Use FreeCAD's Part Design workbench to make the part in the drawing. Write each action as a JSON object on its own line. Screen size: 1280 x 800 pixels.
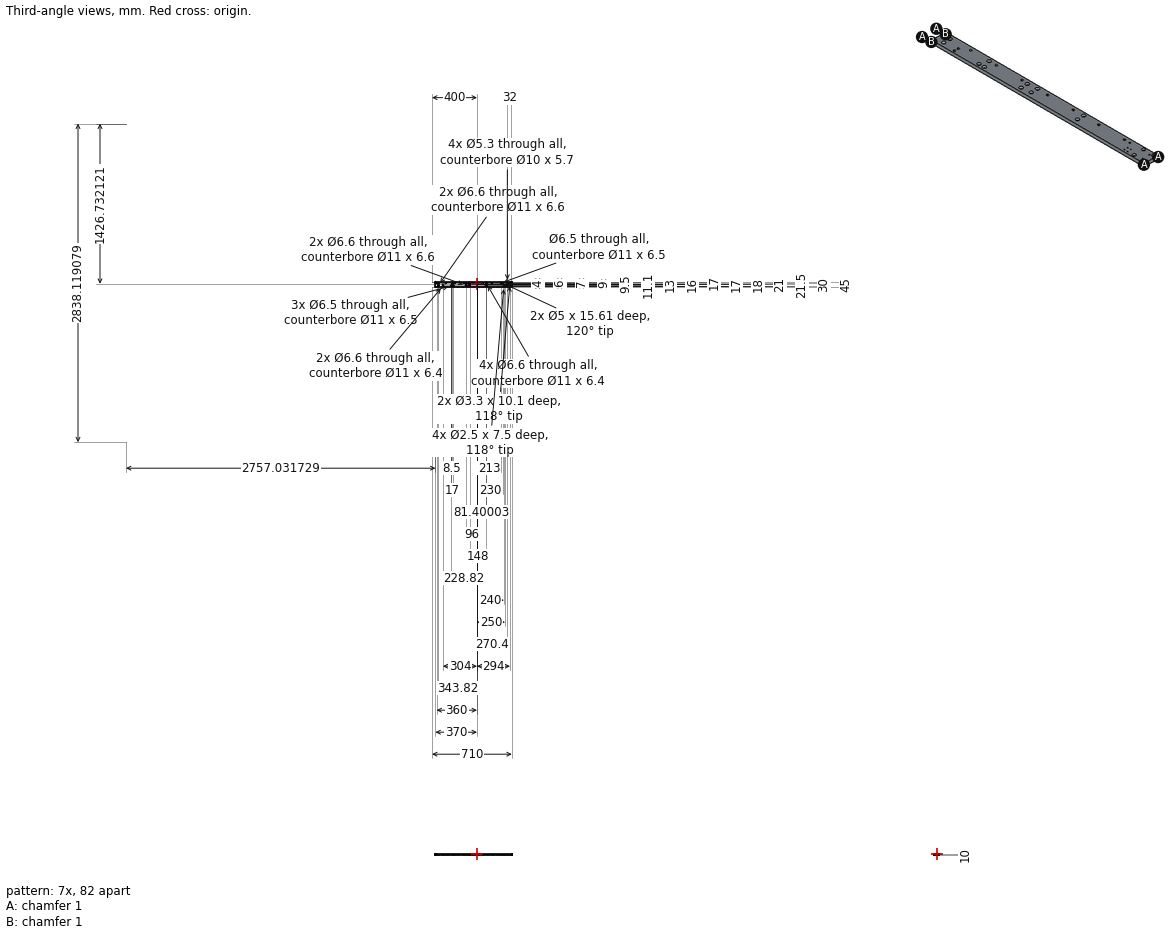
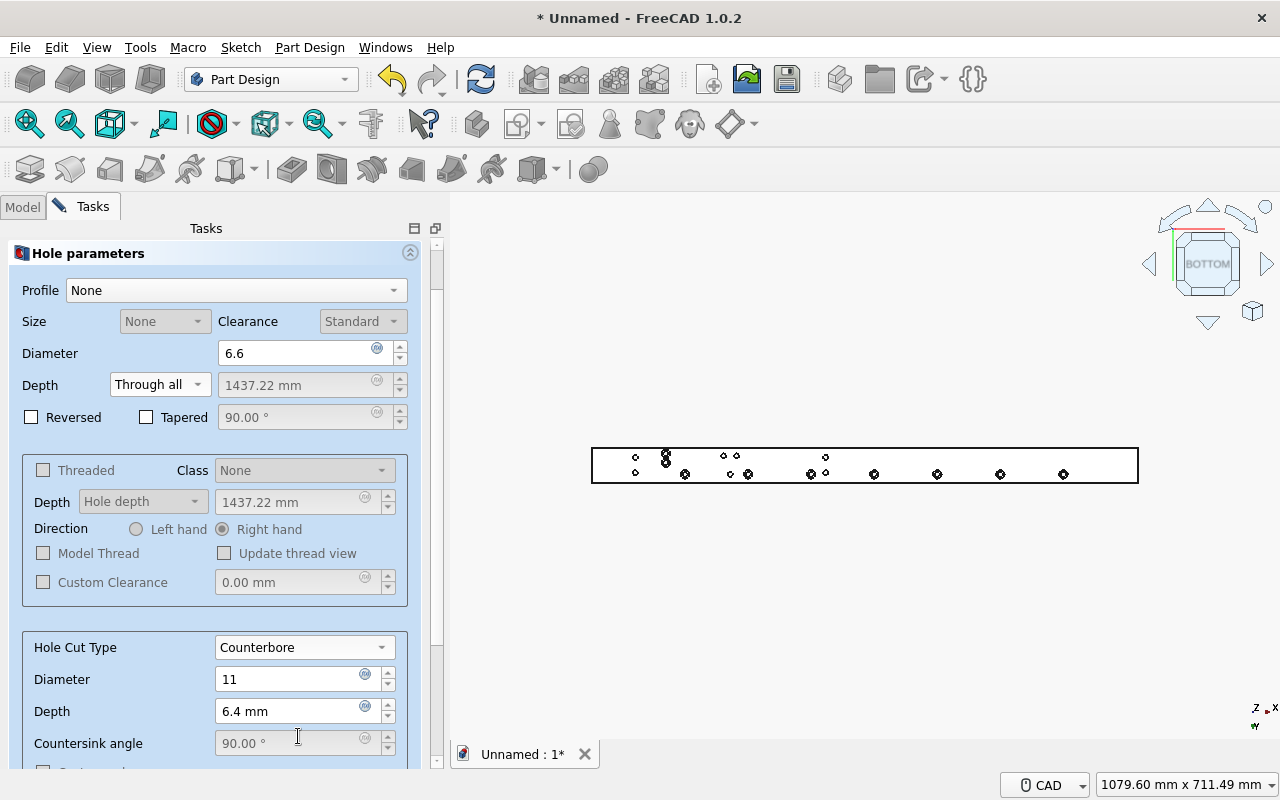
{"action": "scroll", "coordinate": [437, 503], "scroll_direction": "up", "scroll_amount": 2}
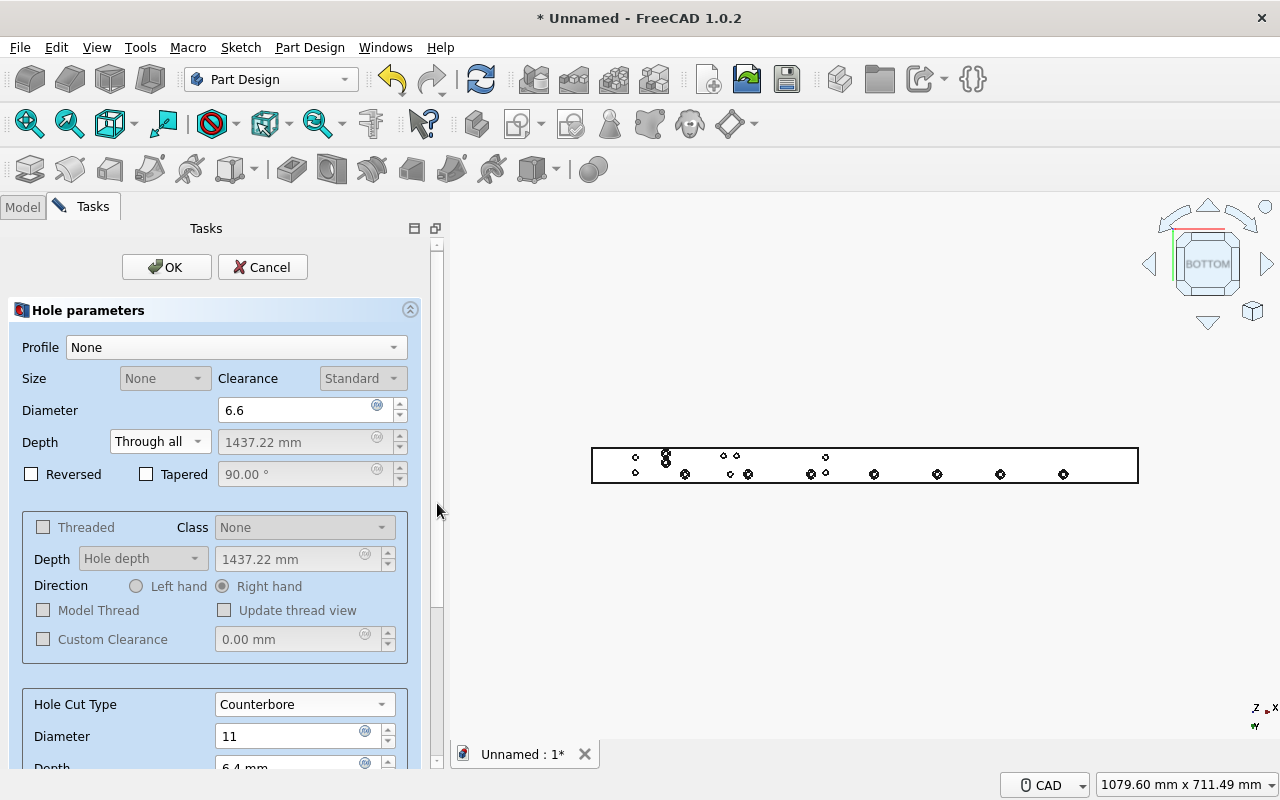
{"action": "left_click", "coordinate": [167, 267]}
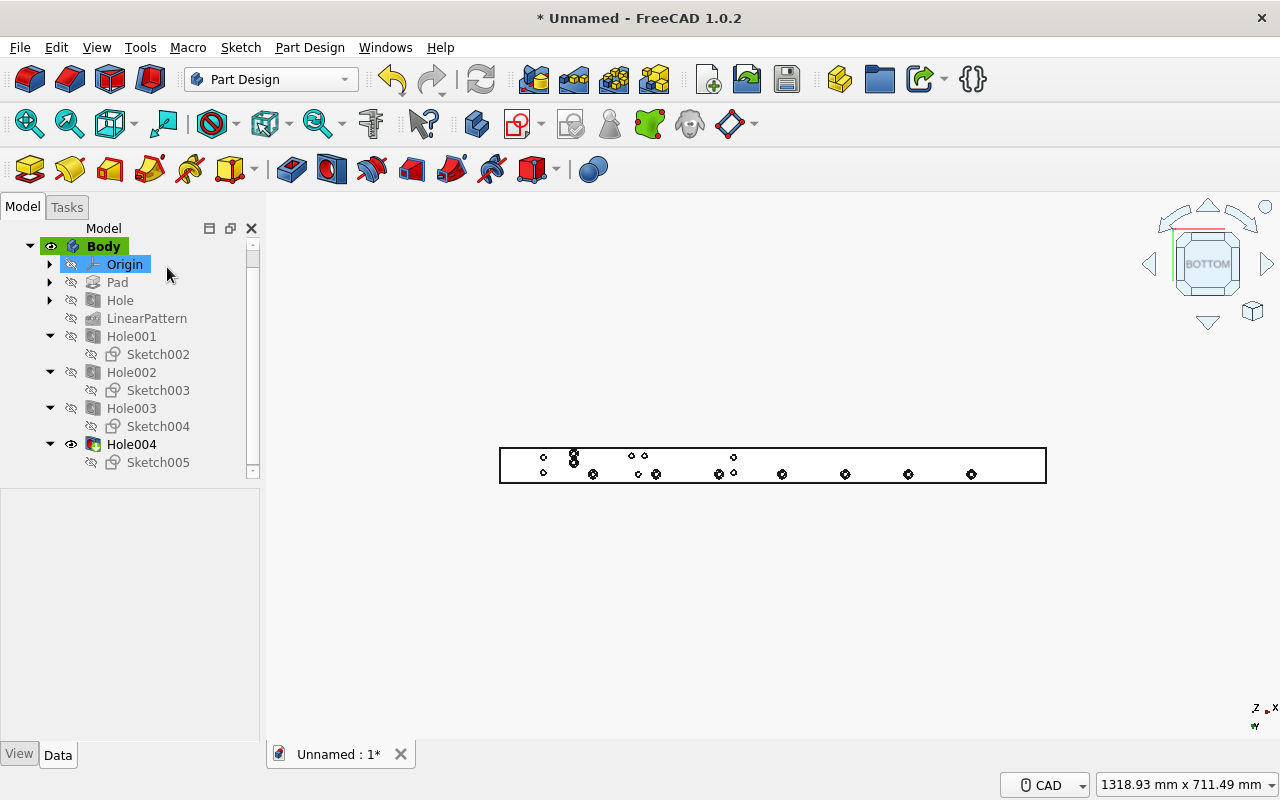
{"action": "key", "text": "0"}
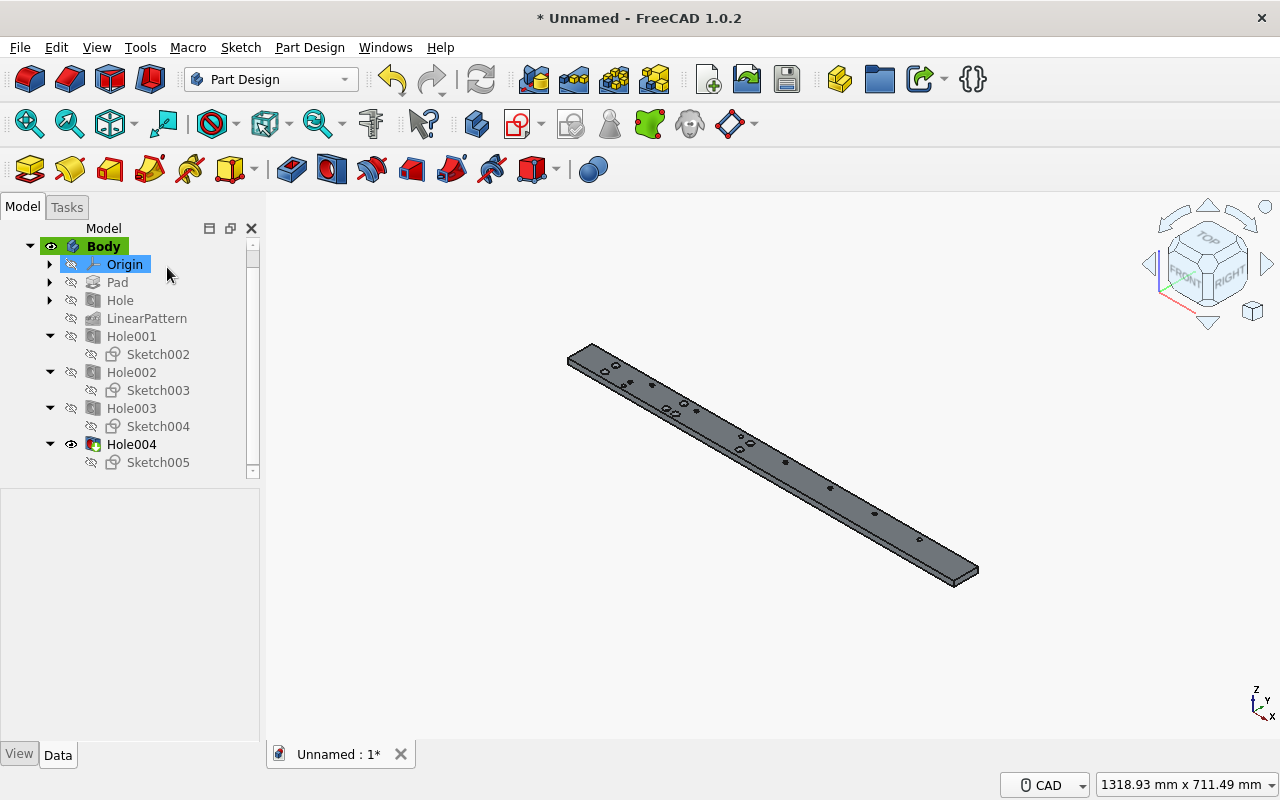
{"action": "left_click", "coordinate": [30, 124]}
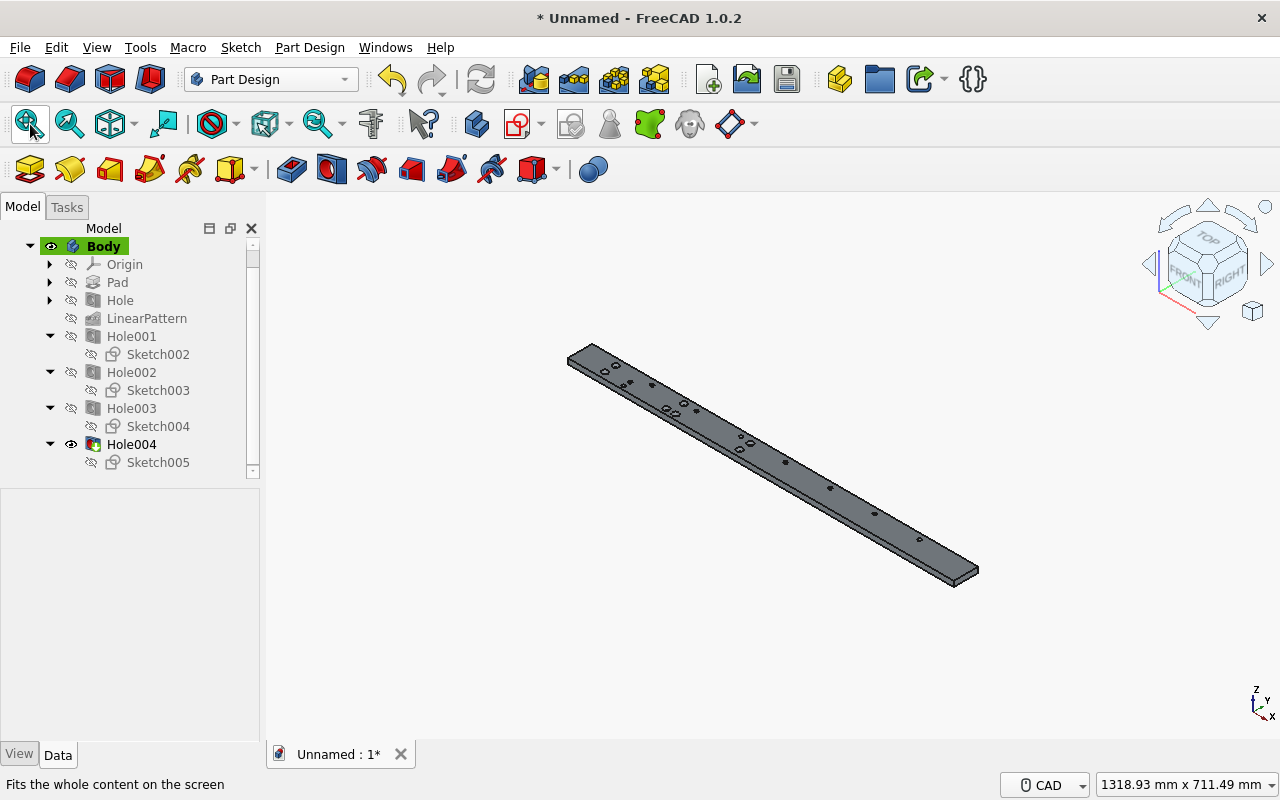
{"action": "left_click", "coordinate": [938, 557]}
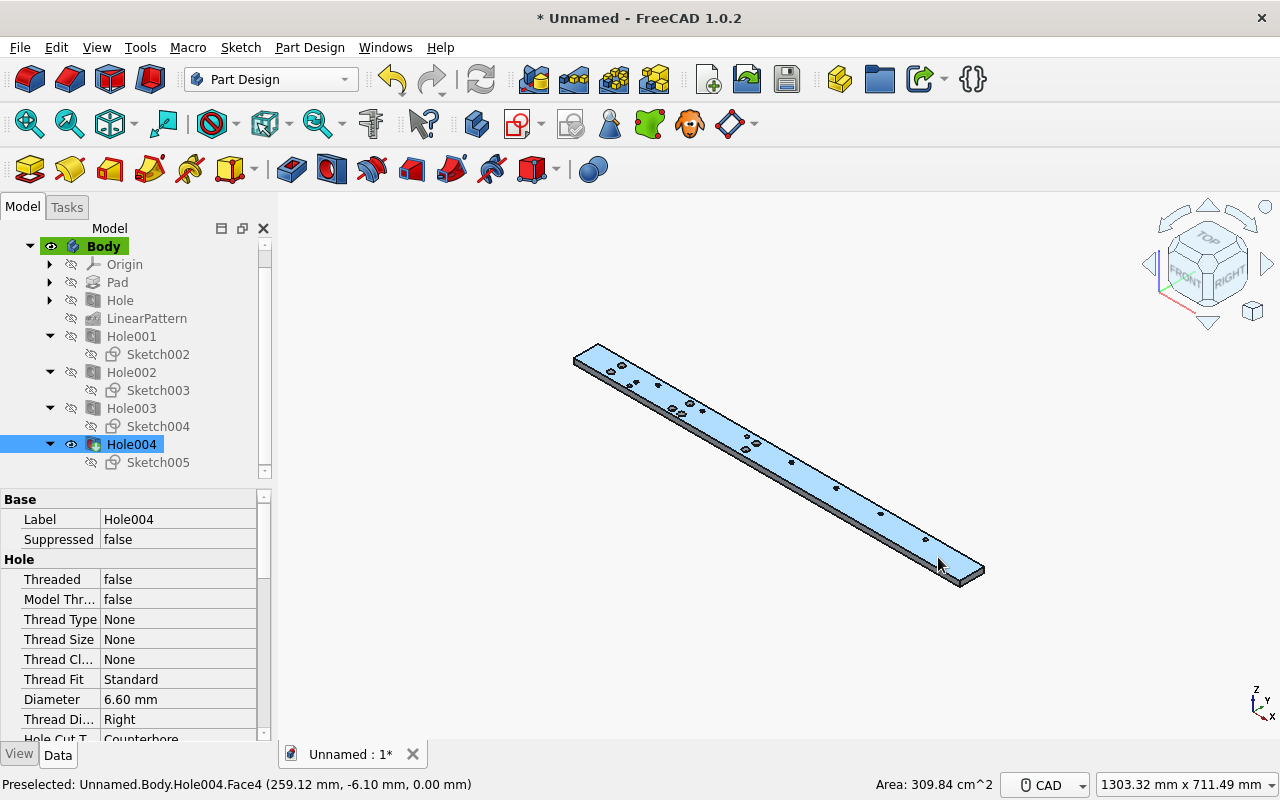
{"action": "left_click", "coordinate": [518, 124]}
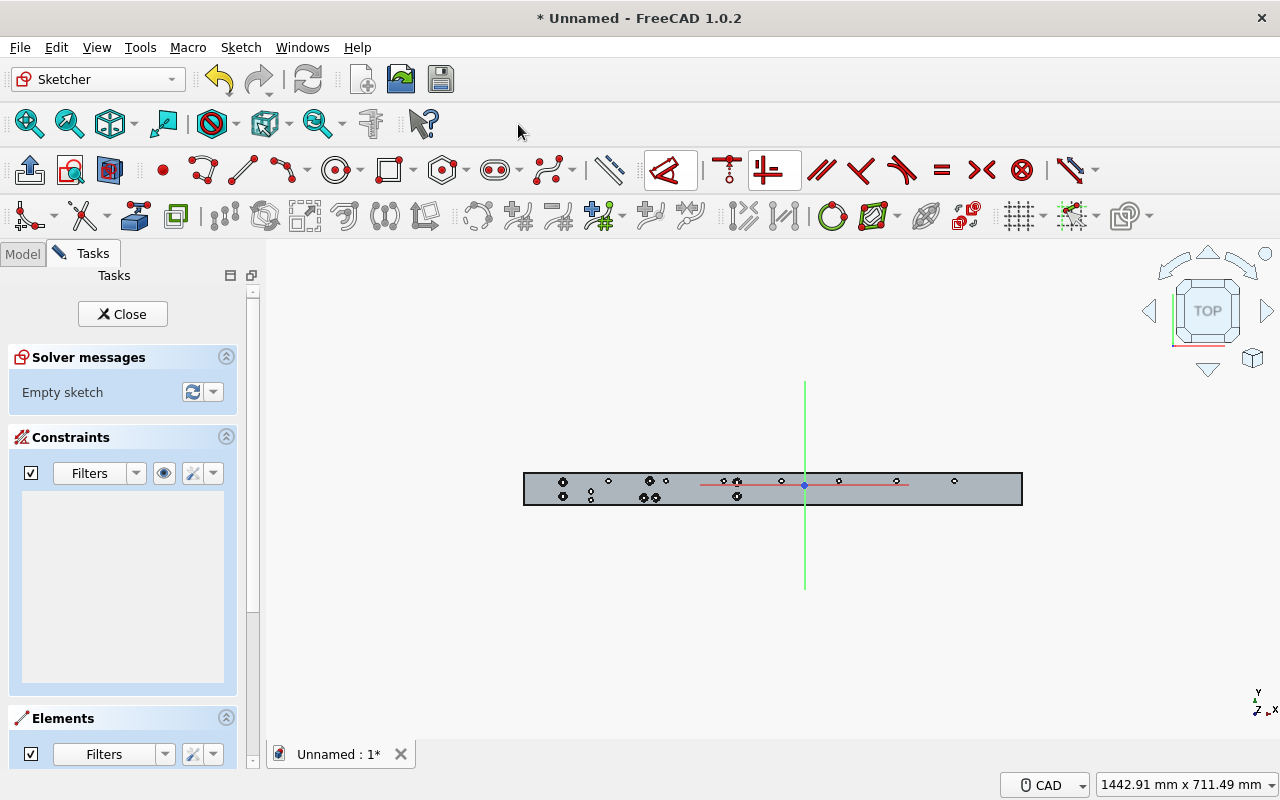
{"action": "scroll", "coordinate": [836, 487], "scroll_direction": "up", "scroll_amount": 8}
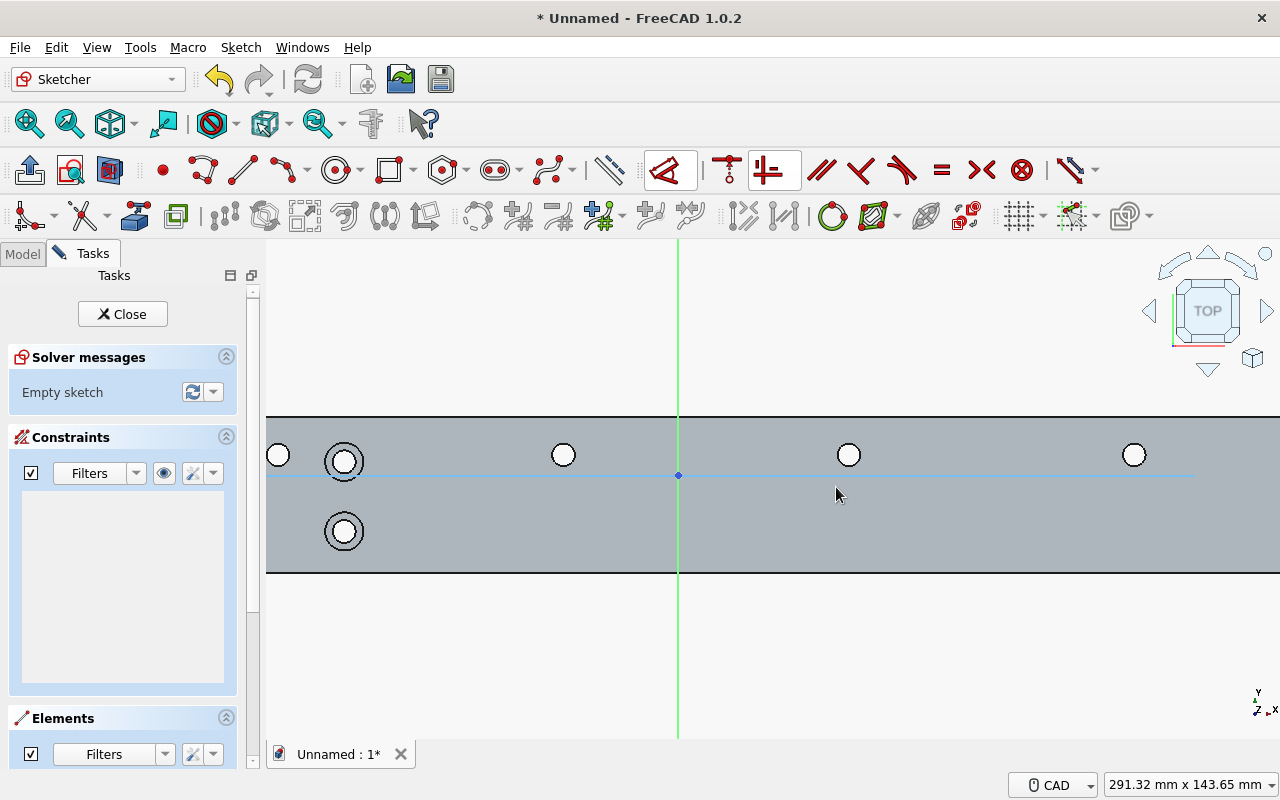
{"action": "left_click", "coordinate": [336, 170]}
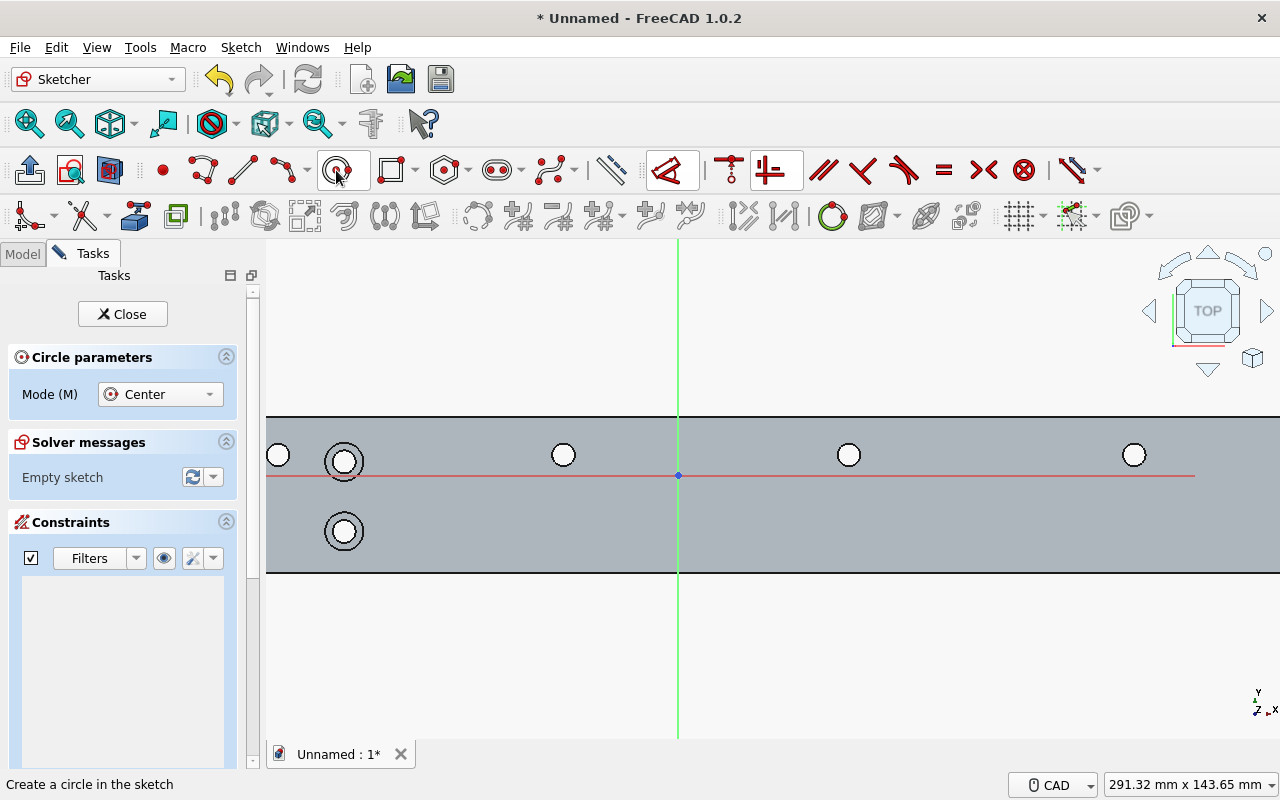
{"action": "scroll", "coordinate": [962, 451], "scroll_direction": "up", "scroll_amount": 4}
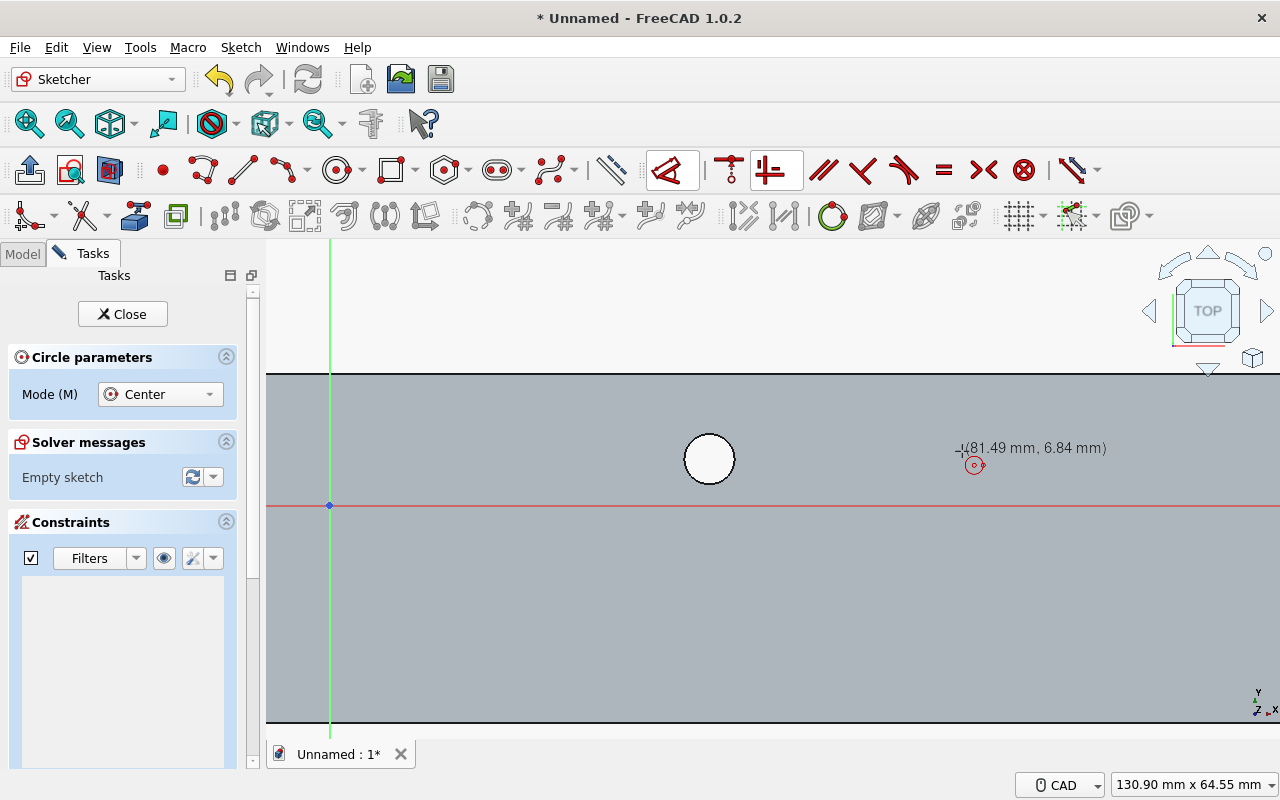
{"action": "left_click", "coordinate": [960, 451]}
{"action": "left_click", "coordinate": [979, 433]}